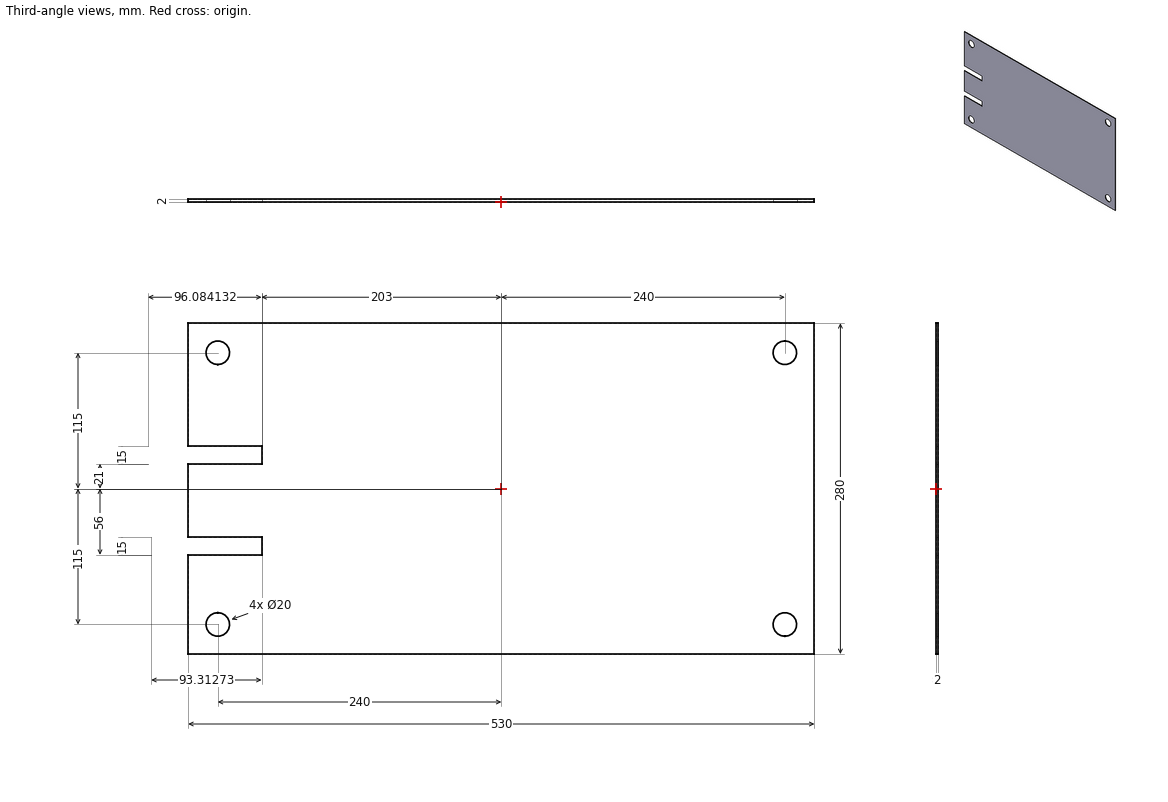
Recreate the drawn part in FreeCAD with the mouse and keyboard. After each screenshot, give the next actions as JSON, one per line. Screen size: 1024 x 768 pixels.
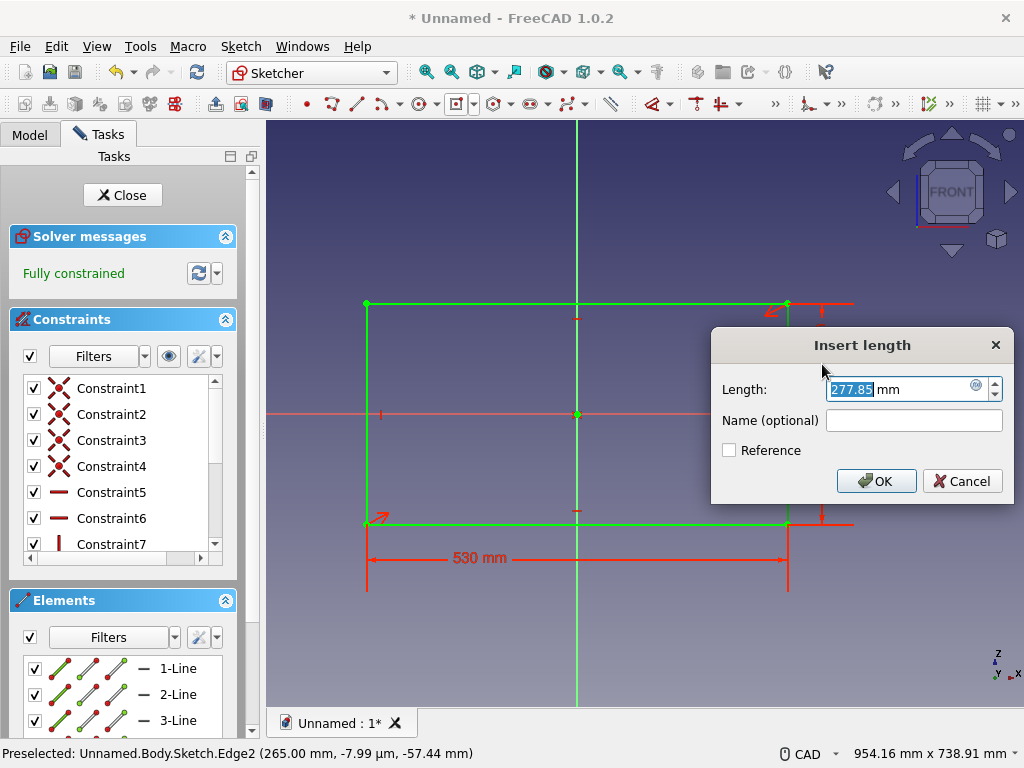
{"action": "type", "text": "280"}
{"action": "key", "text": "Return"}
{"action": "key", "text": "Escape"}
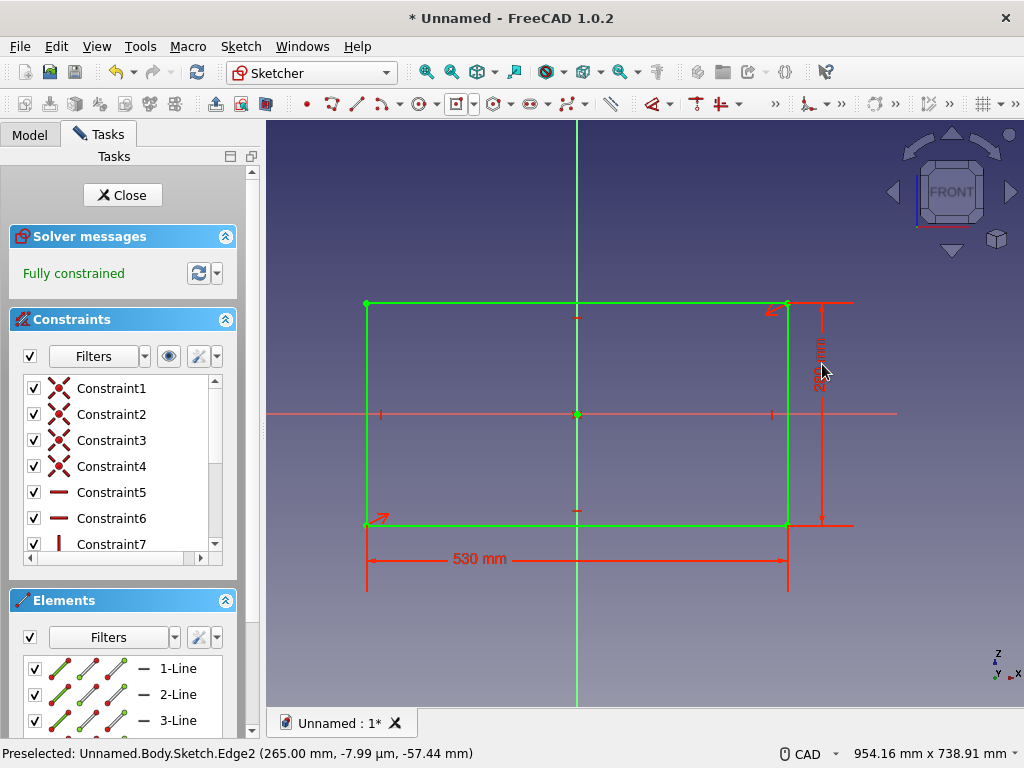
{"action": "left_click", "coordinate": [123, 195]}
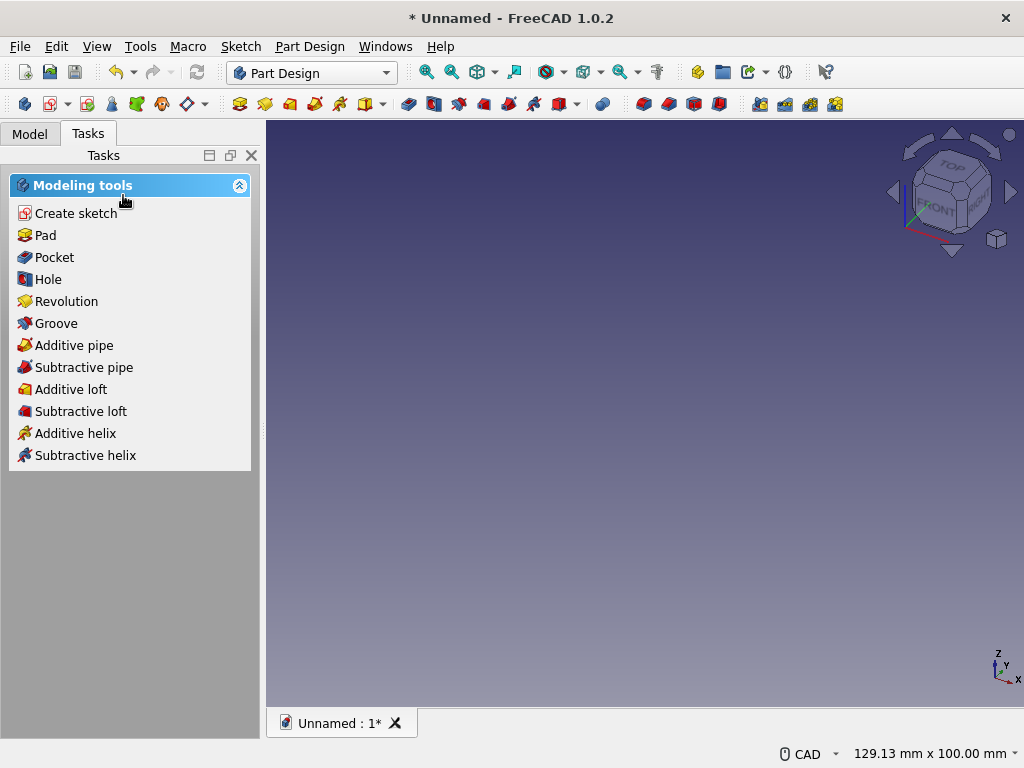
{"action": "left_click", "coordinate": [240, 104]}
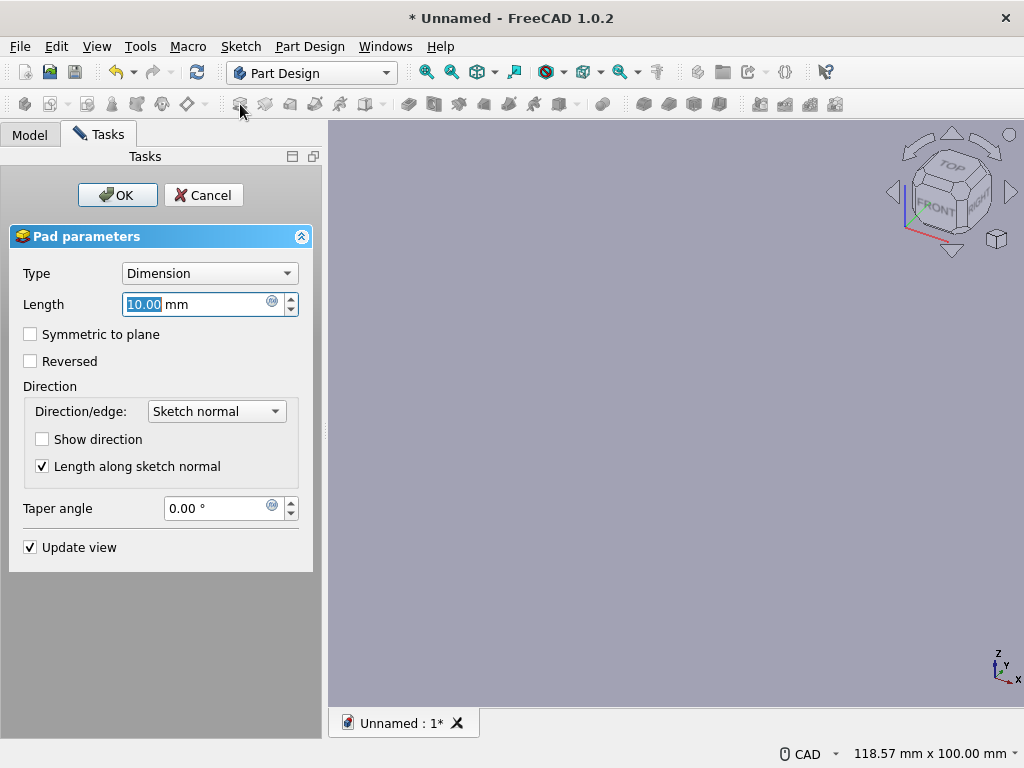
{"action": "type", "text": "2"}
{"action": "key", "text": "Tab"}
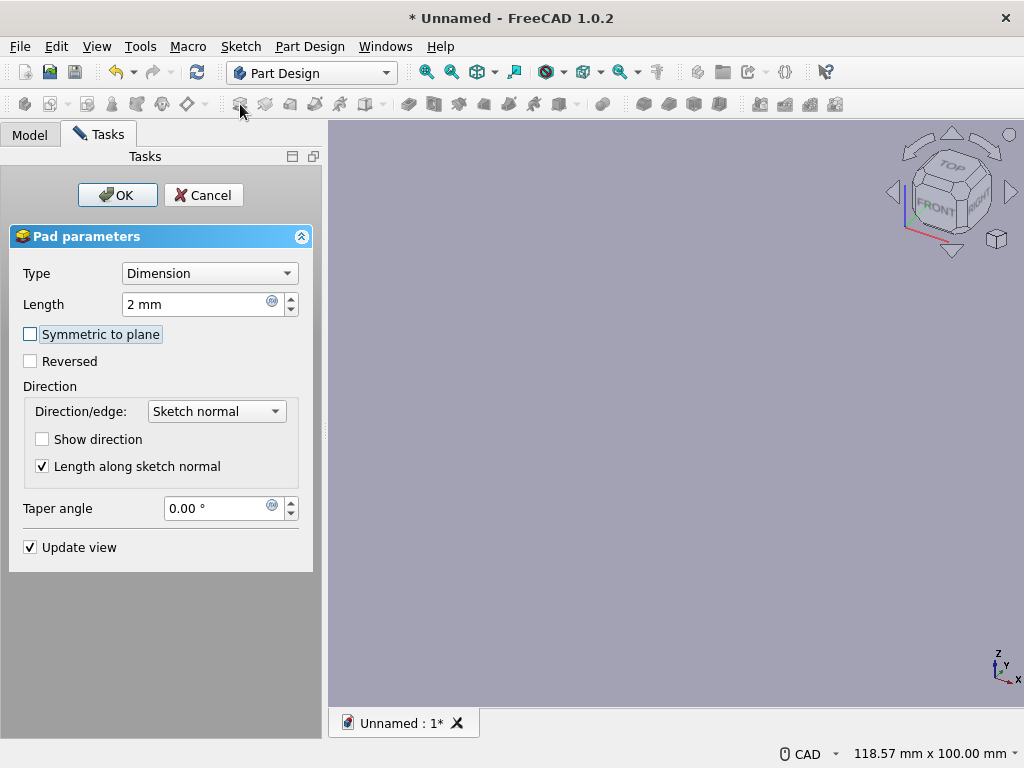
{"action": "left_click", "coordinate": [31, 361]}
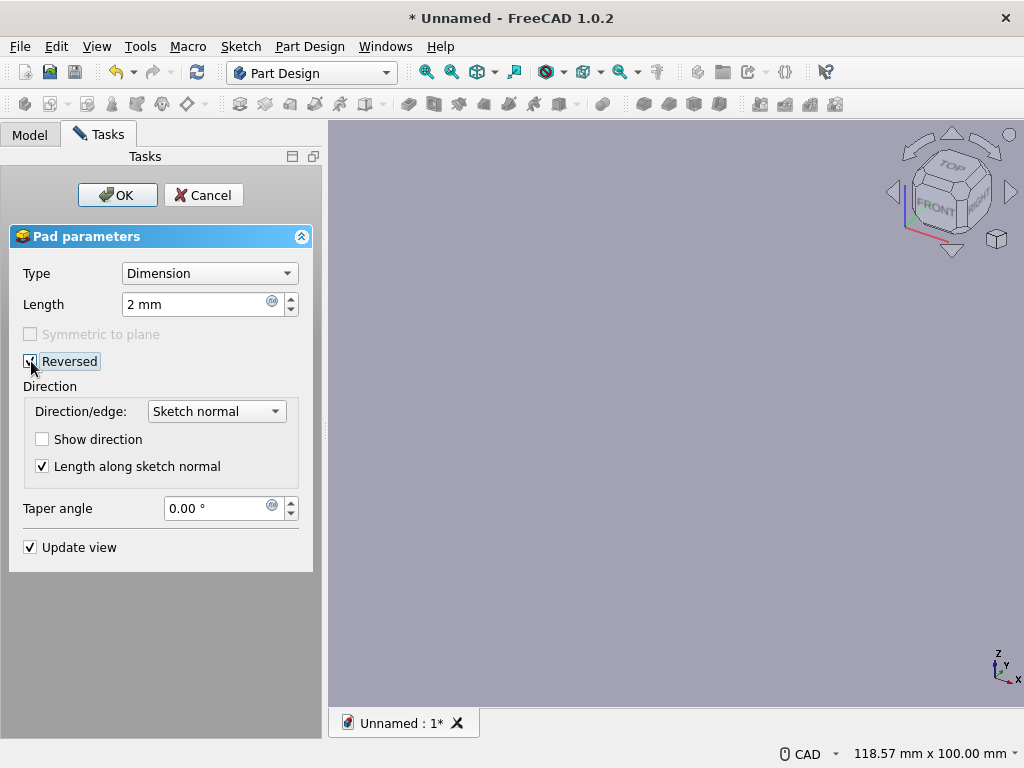
{"action": "left_click", "coordinate": [118, 195]}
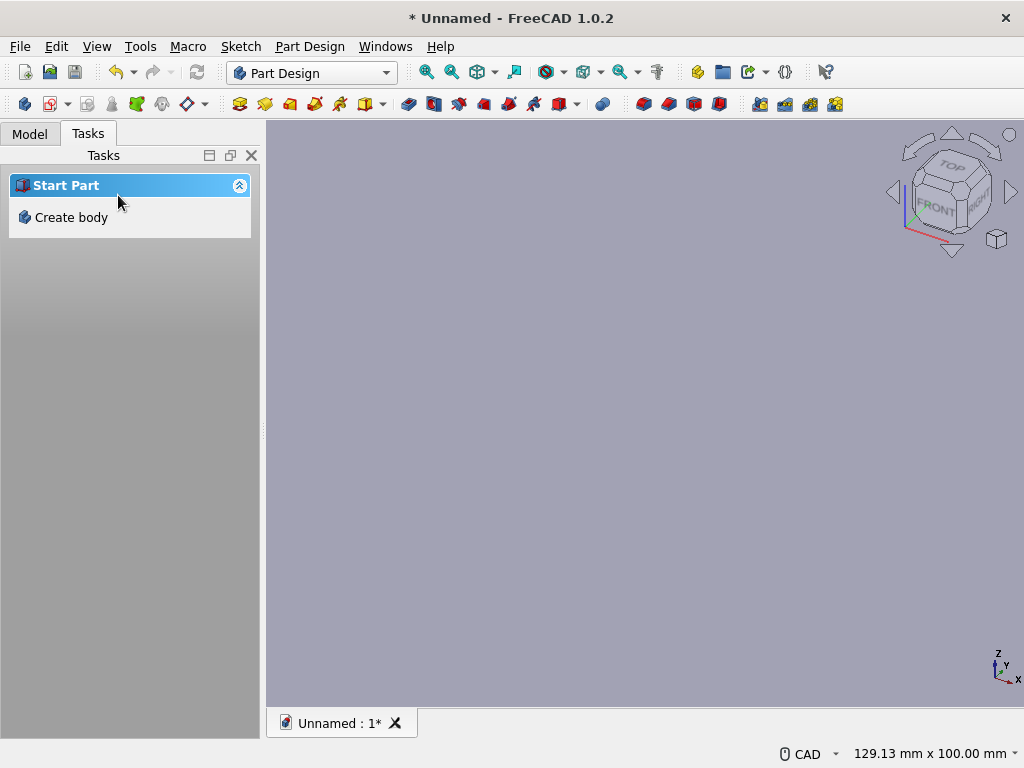
{"action": "left_click", "coordinate": [427, 72]}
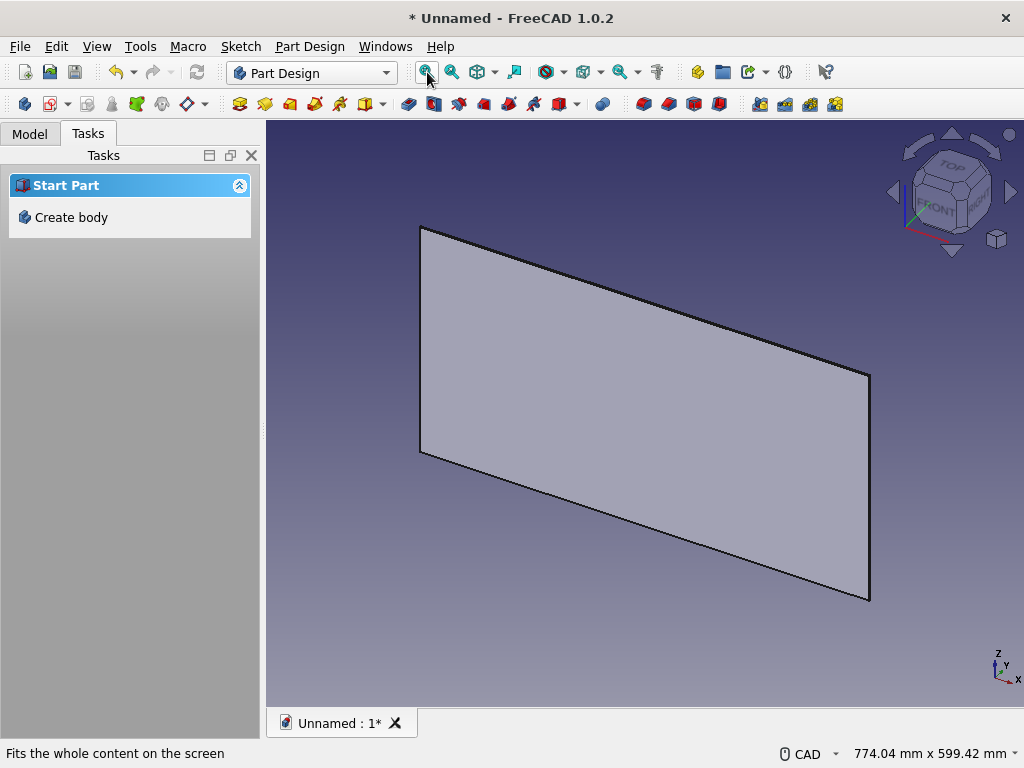
{"action": "key", "text": "4"}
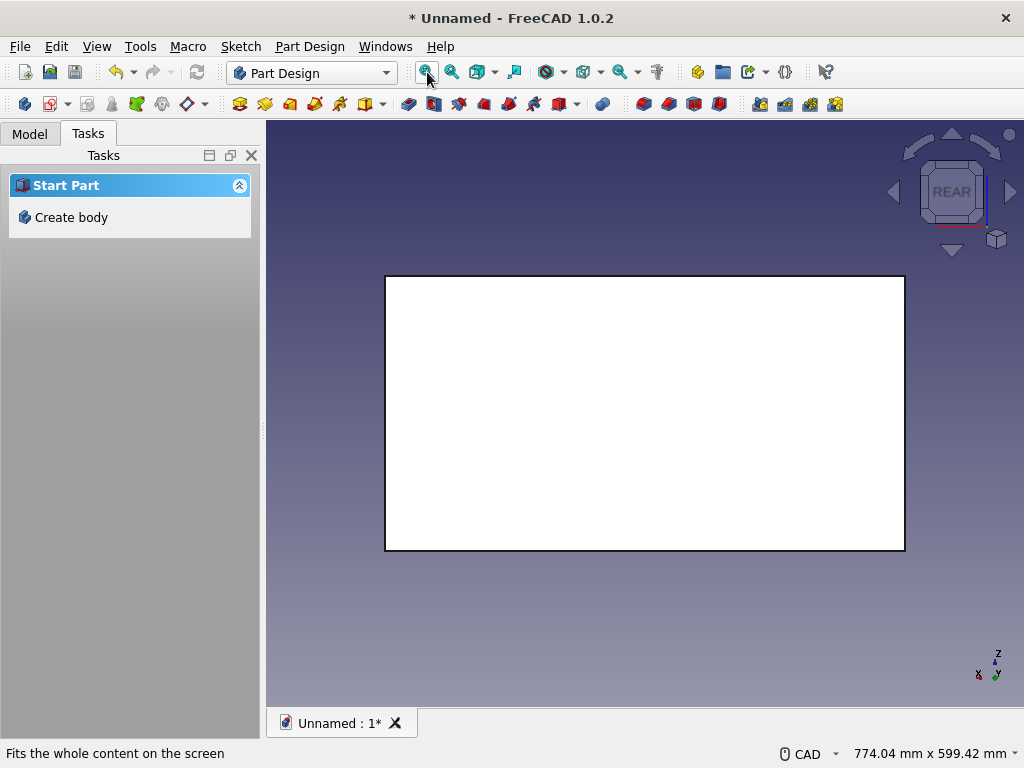
{"action": "left_click", "coordinate": [571, 412]}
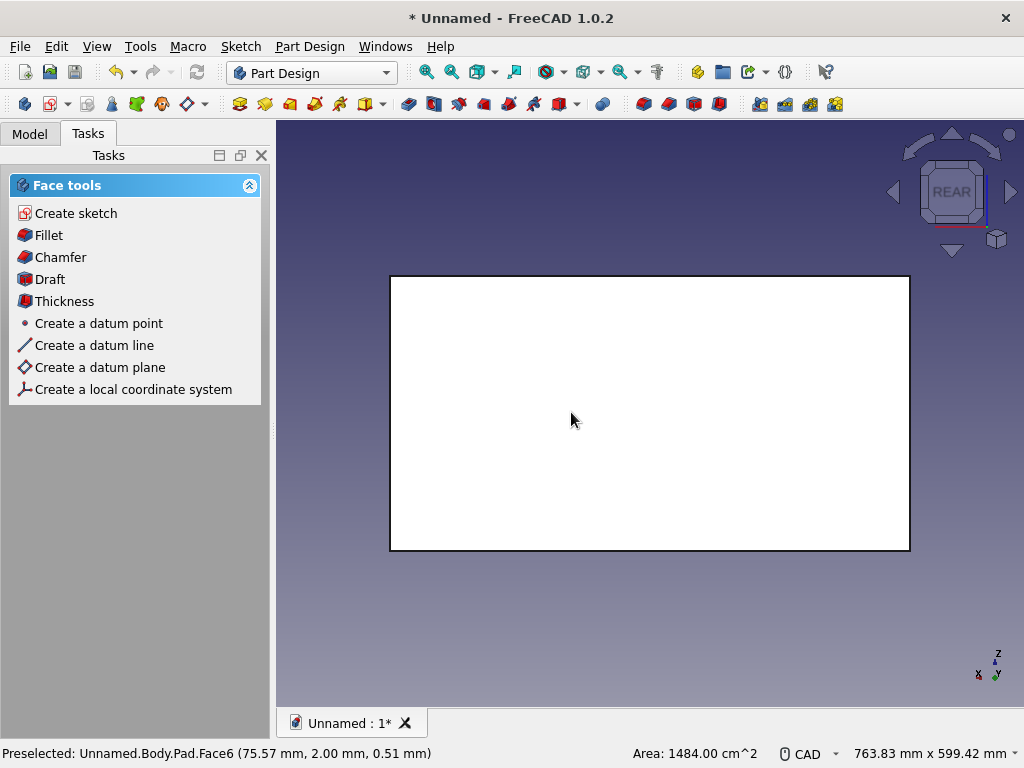
{"action": "left_click", "coordinate": [50, 104]}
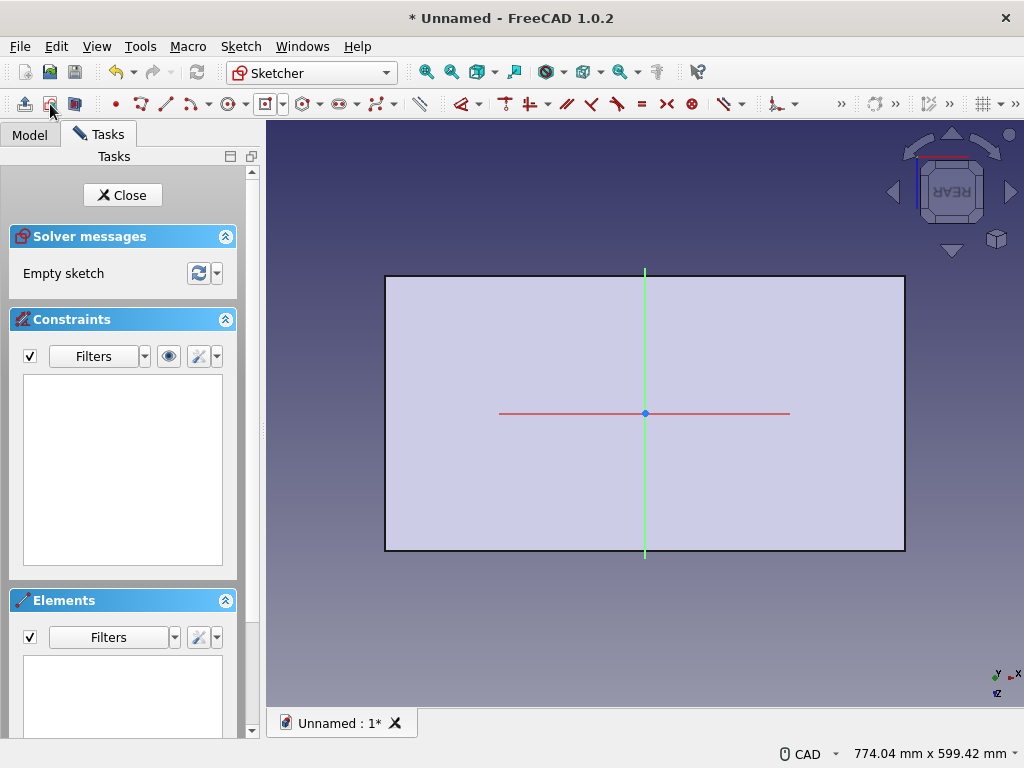
{"action": "scroll", "coordinate": [294, 413], "scroll_direction": "down", "scroll_amount": 1}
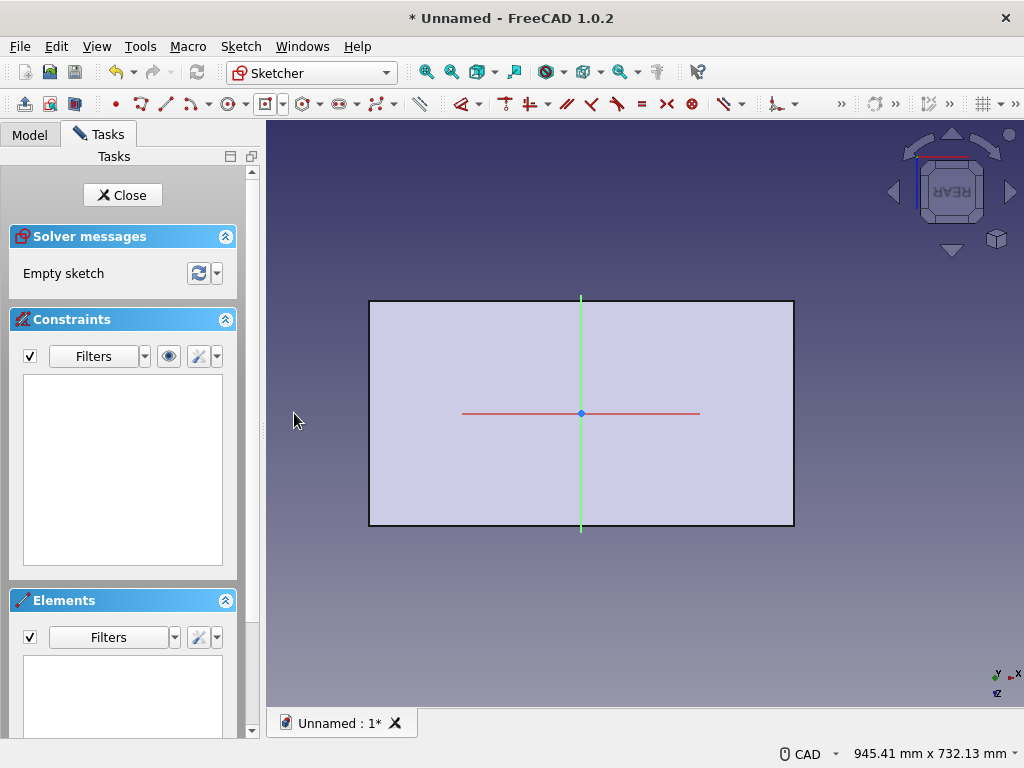
{"action": "left_click", "coordinate": [228, 104]}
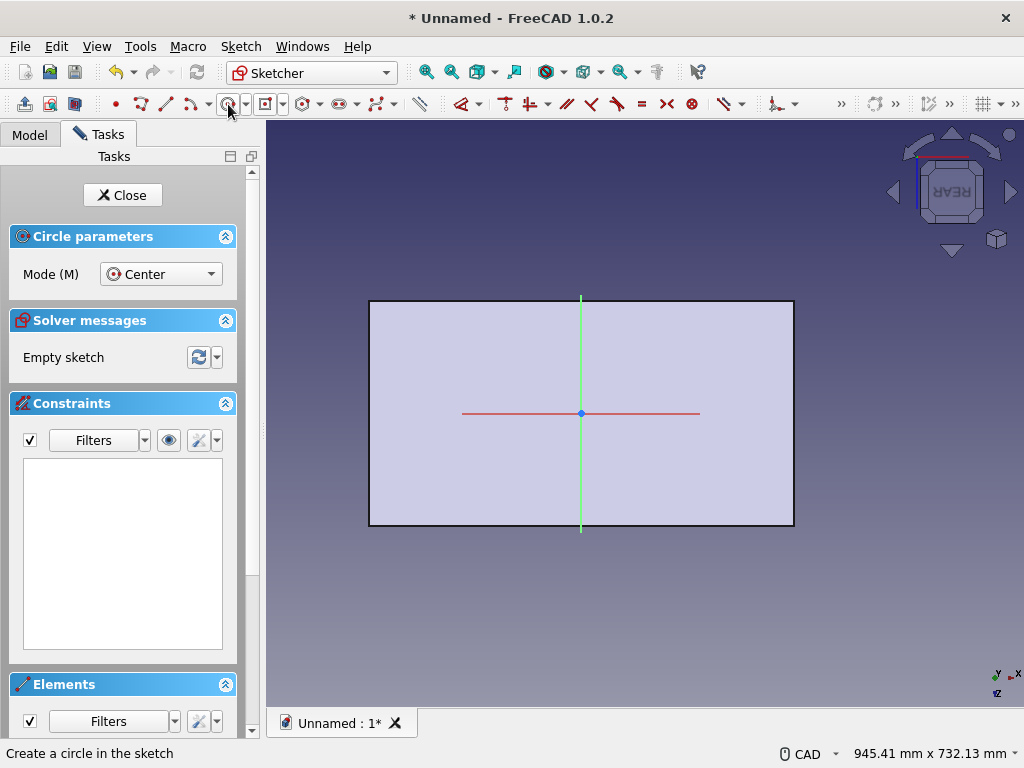
{"action": "scroll", "coordinate": [389, 321], "scroll_direction": "up", "scroll_amount": 6}